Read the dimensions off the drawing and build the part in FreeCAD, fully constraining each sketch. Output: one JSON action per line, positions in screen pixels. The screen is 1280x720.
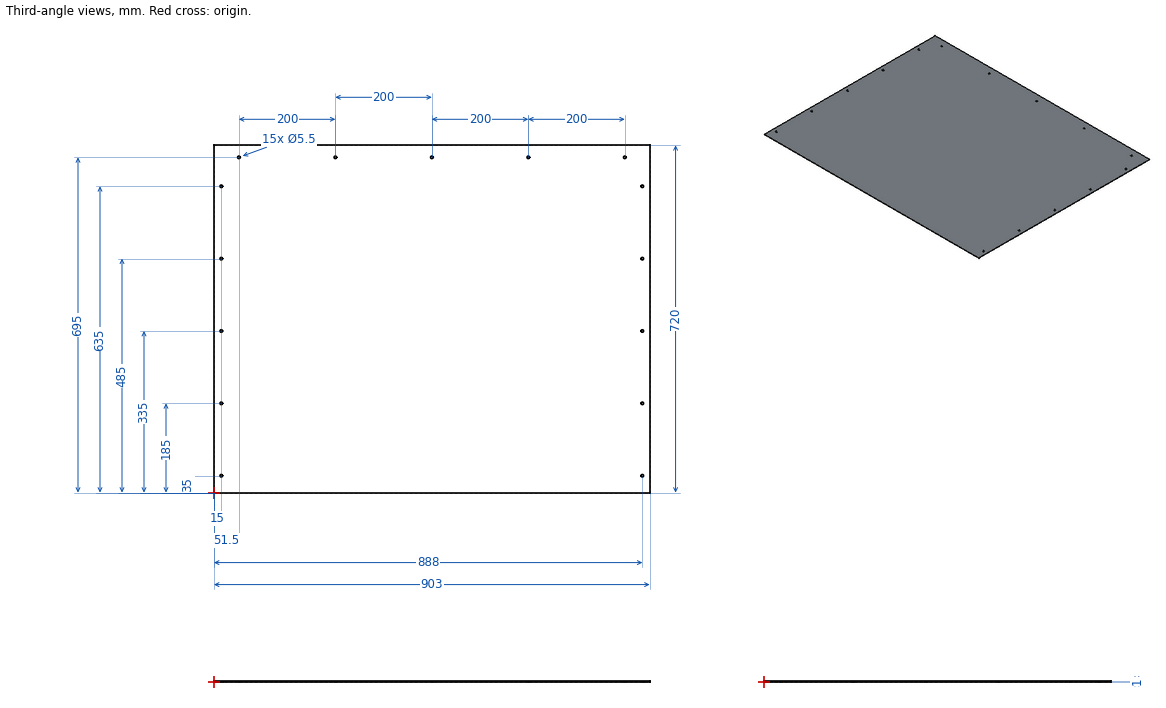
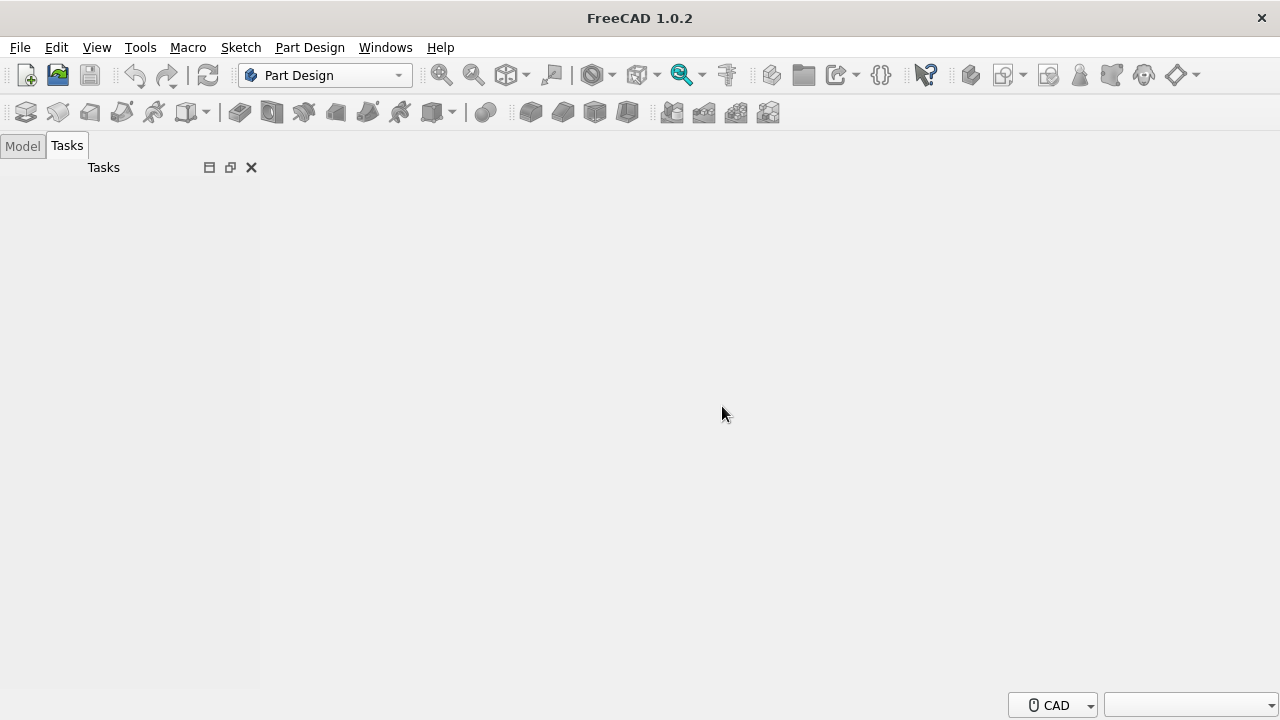
{"action": "key", "text": "ctrl+n"}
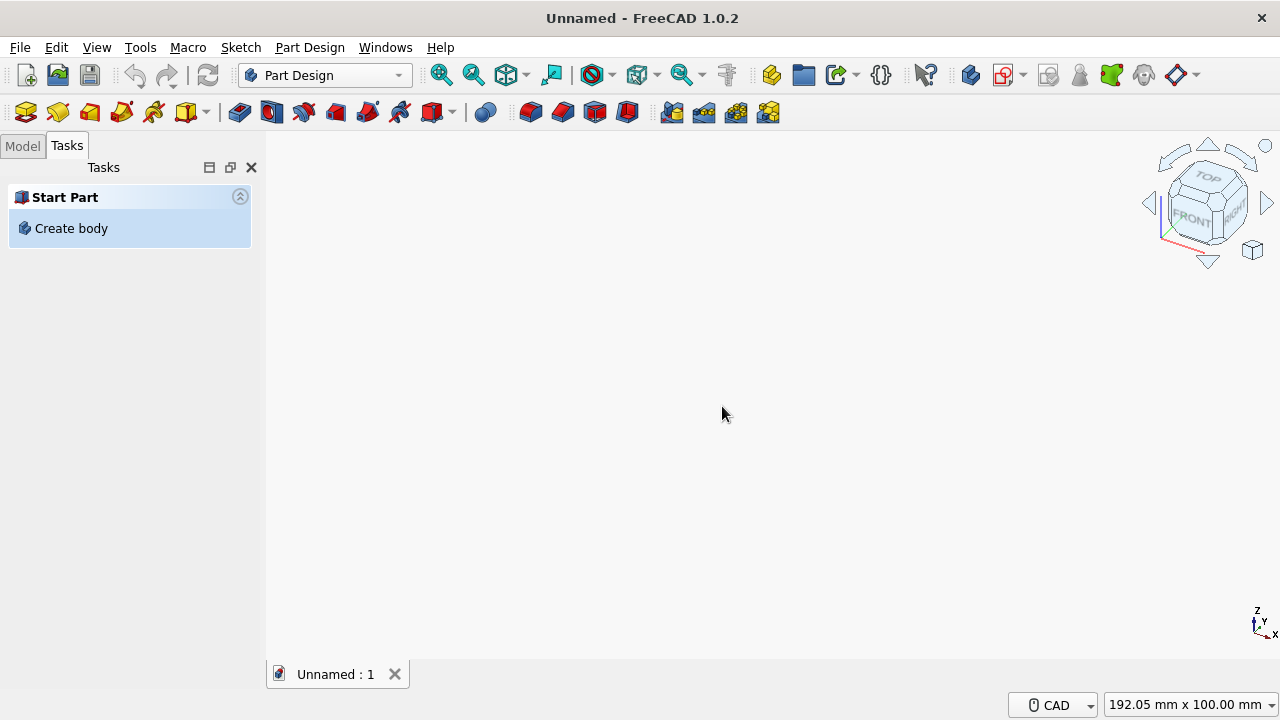
{"action": "left_click", "coordinate": [1004, 76]}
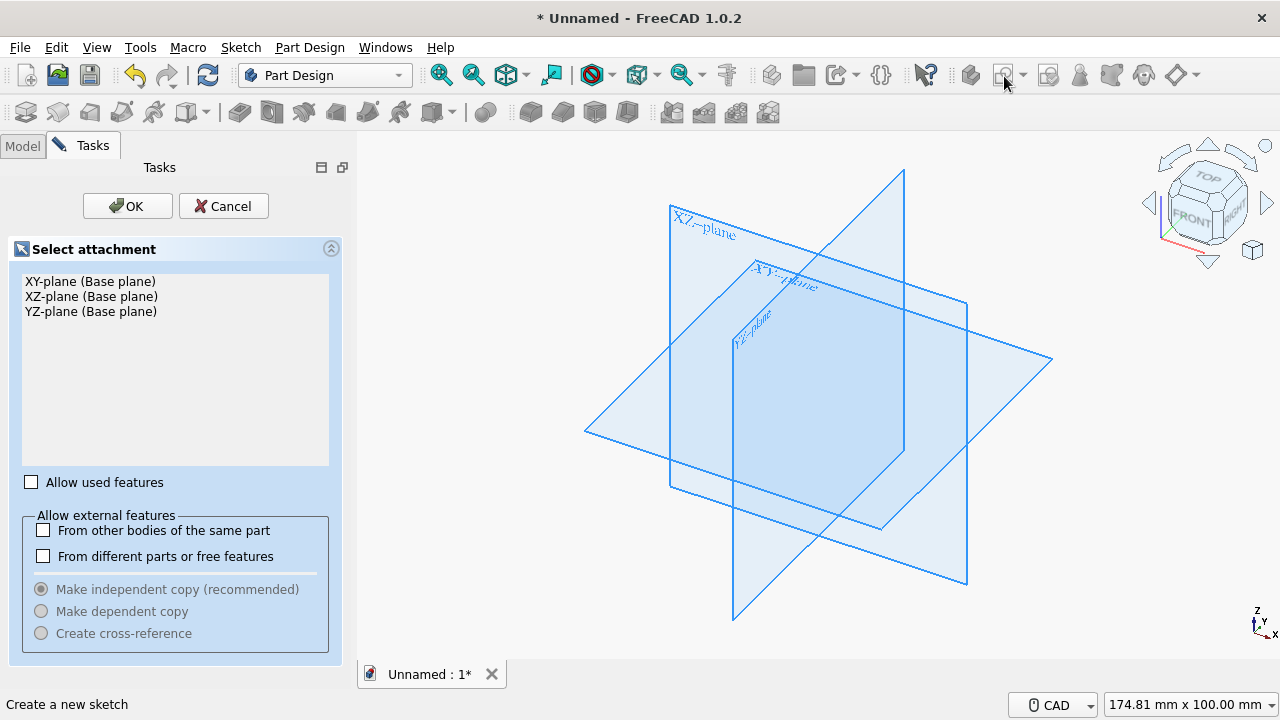
{"action": "left_click", "coordinate": [82, 282]}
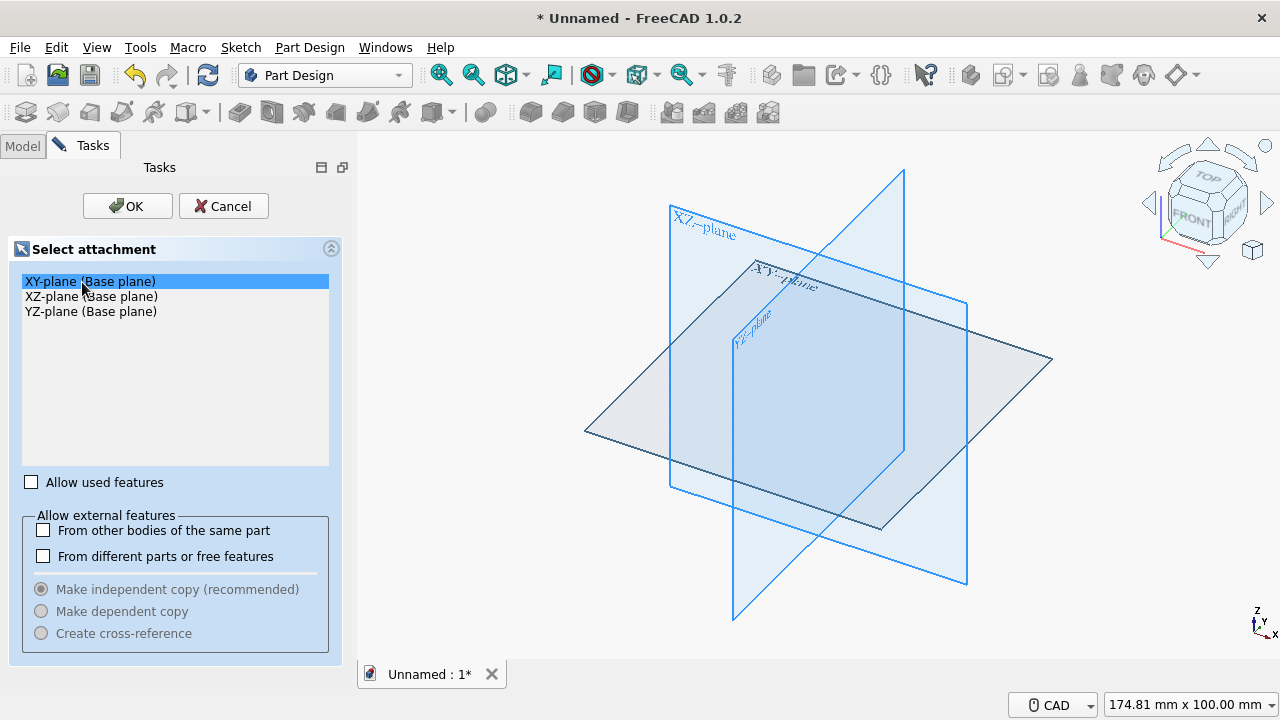
{"action": "left_click", "coordinate": [128, 206]}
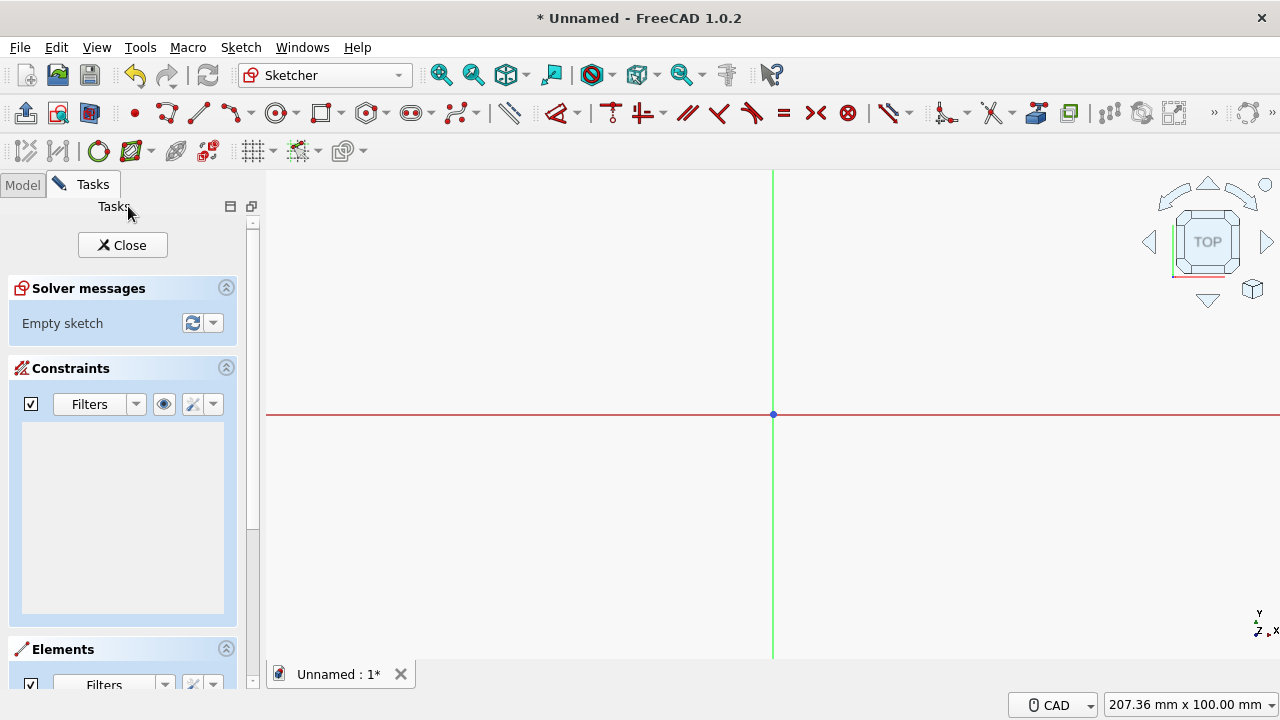
{"action": "scroll", "coordinate": [477, 590], "scroll_direction": "down", "scroll_amount": 12}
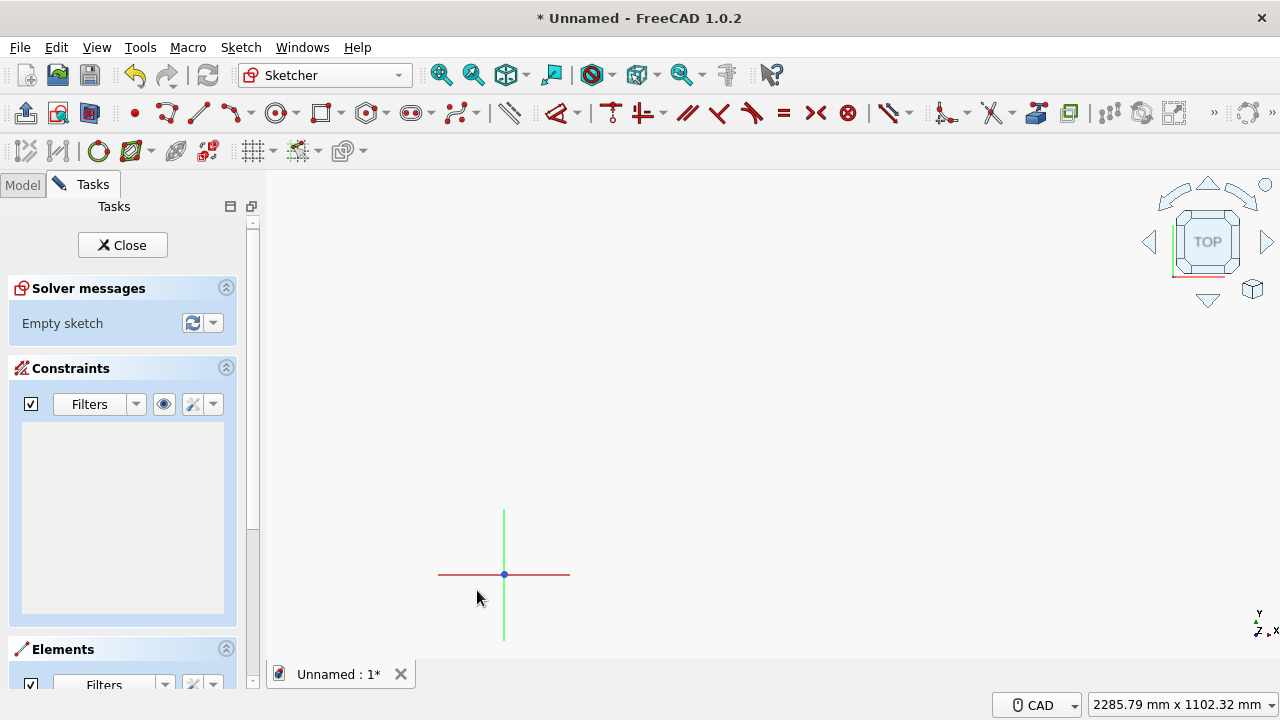
{"action": "key", "text": "g r"}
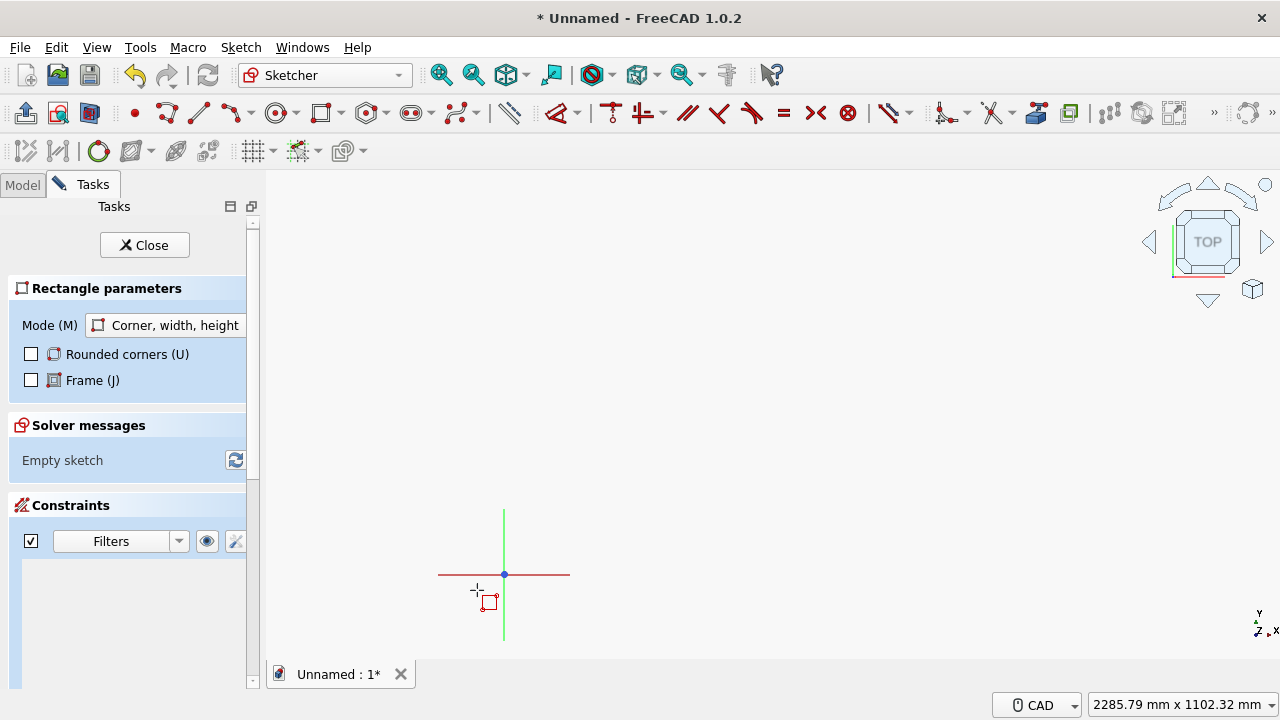
{"action": "left_click", "coordinate": [504, 575]}
{"action": "left_click", "coordinate": [905, 255]}
{"action": "key", "text": "Escape"}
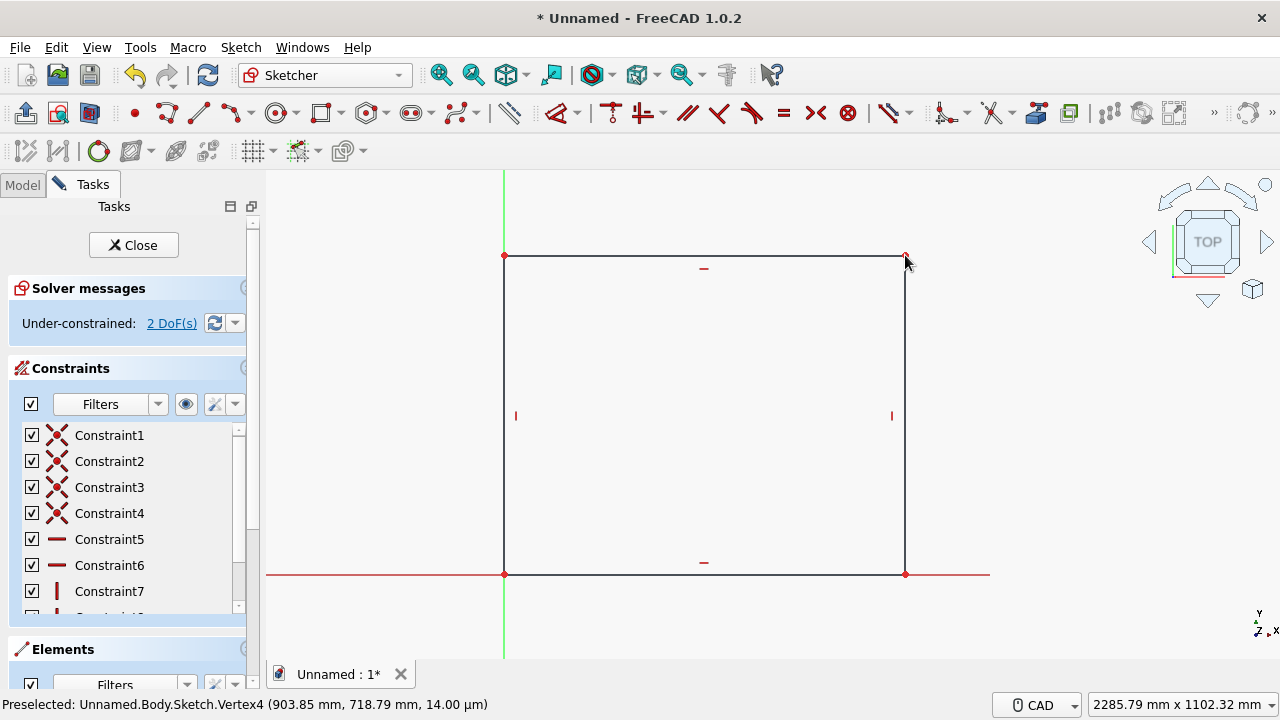
{"action": "key", "text": "d"}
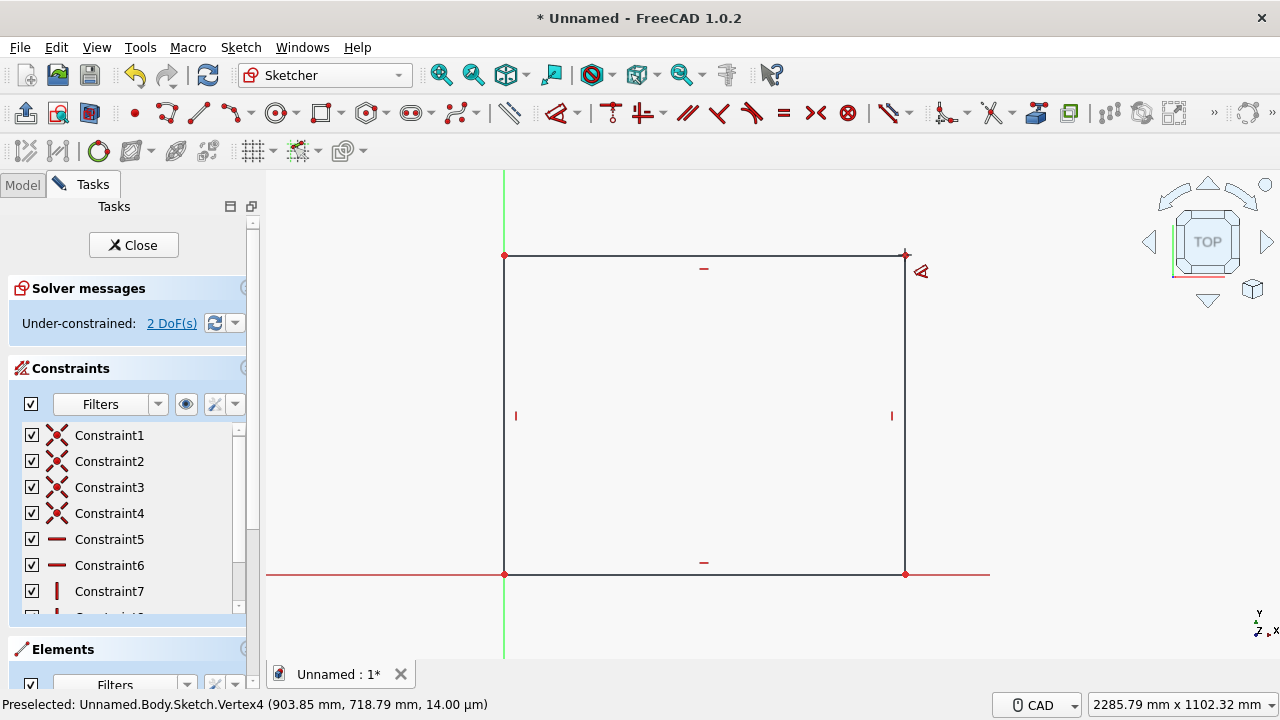
{"action": "left_click", "coordinate": [624, 575]}
{"action": "left_click", "coordinate": [705, 609]}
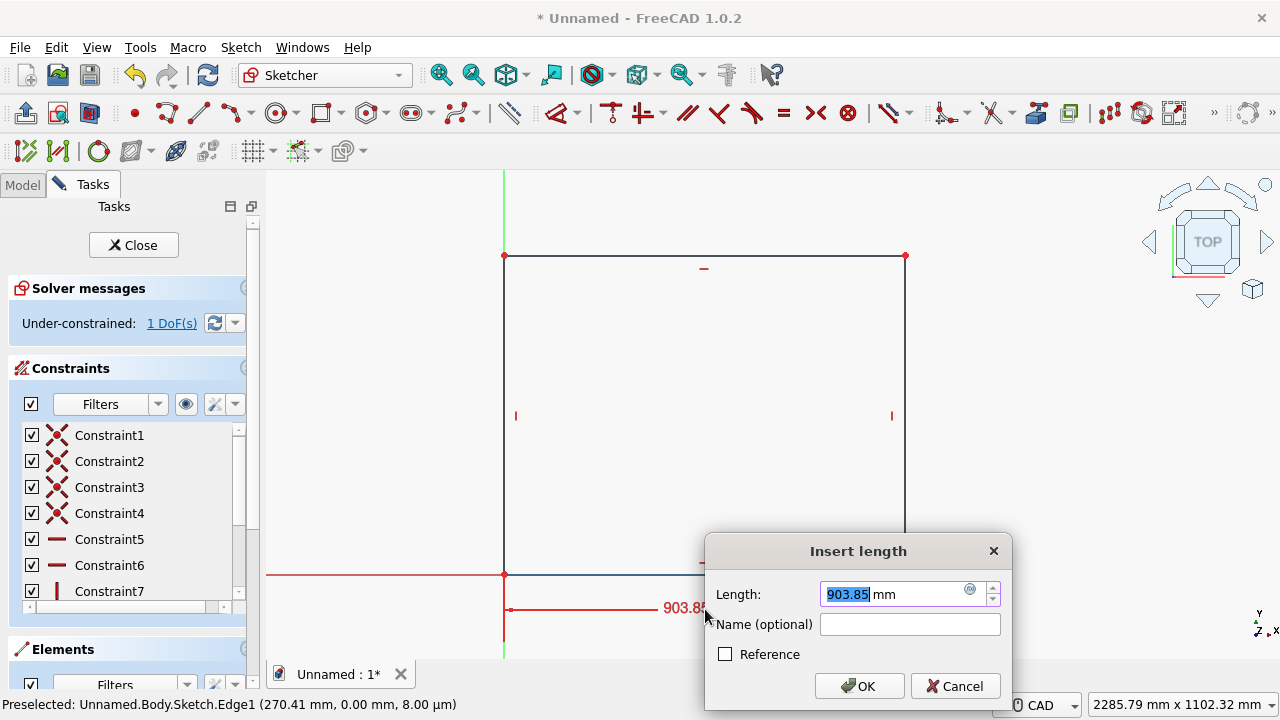
{"action": "type", "text": "903"}
{"action": "key", "text": "Return"}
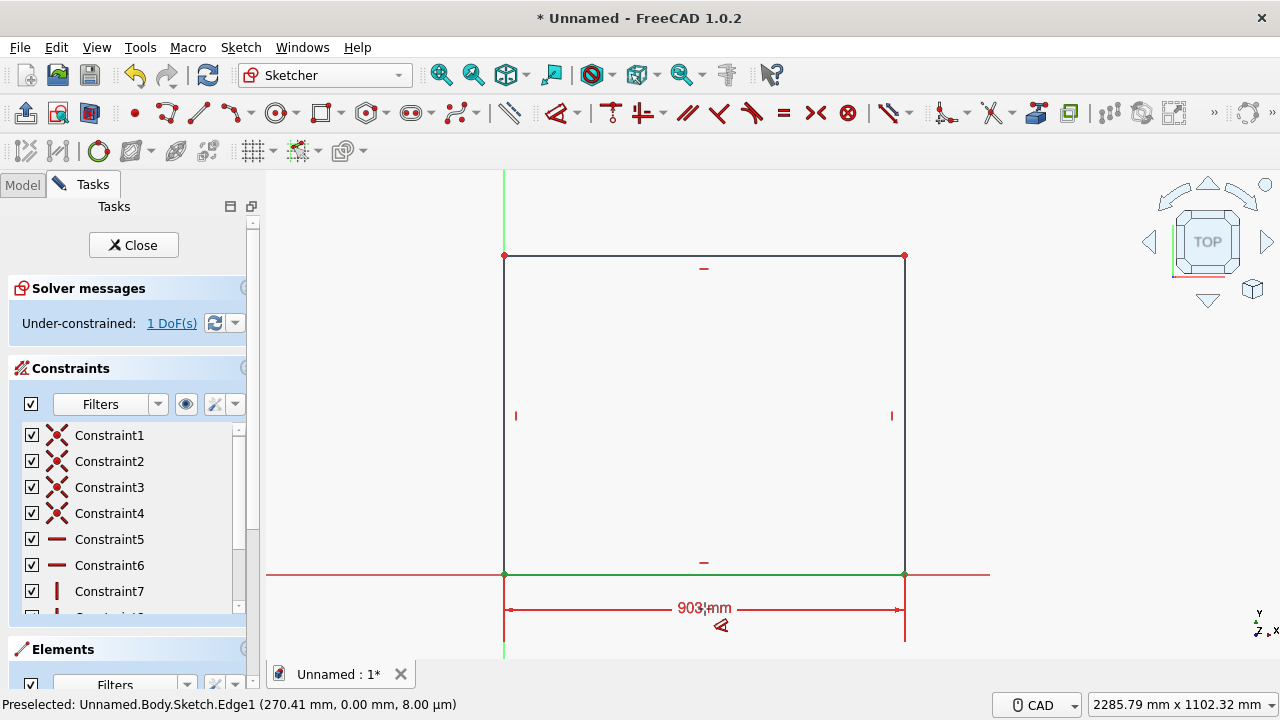
{"action": "left_click", "coordinate": [905, 479]}
{"action": "left_click", "coordinate": [939, 415]}